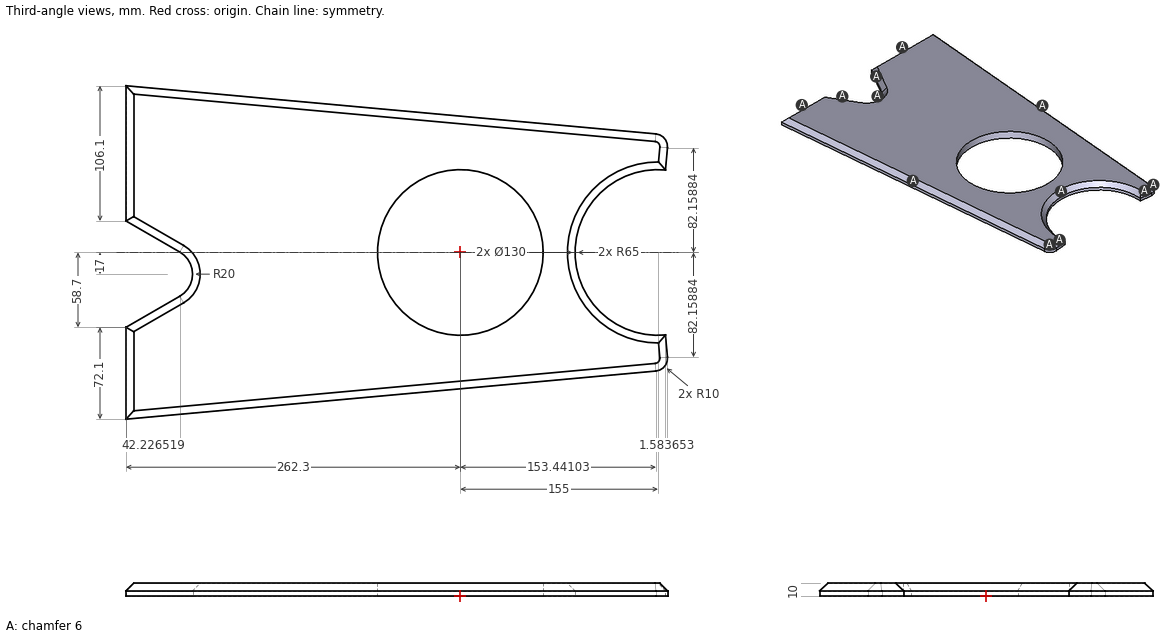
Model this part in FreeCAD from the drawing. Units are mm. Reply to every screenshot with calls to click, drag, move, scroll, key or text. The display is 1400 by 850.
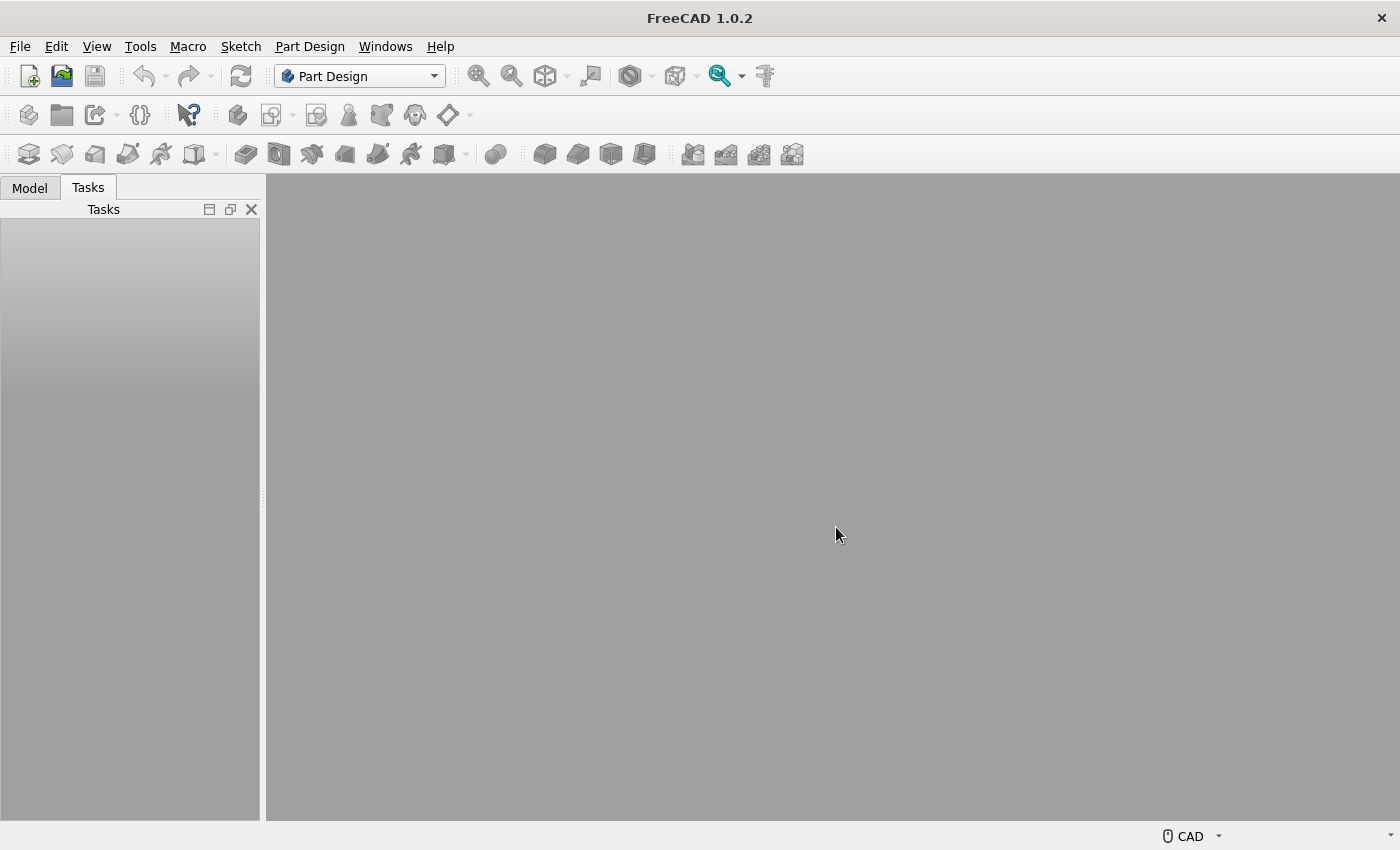
click(29, 76)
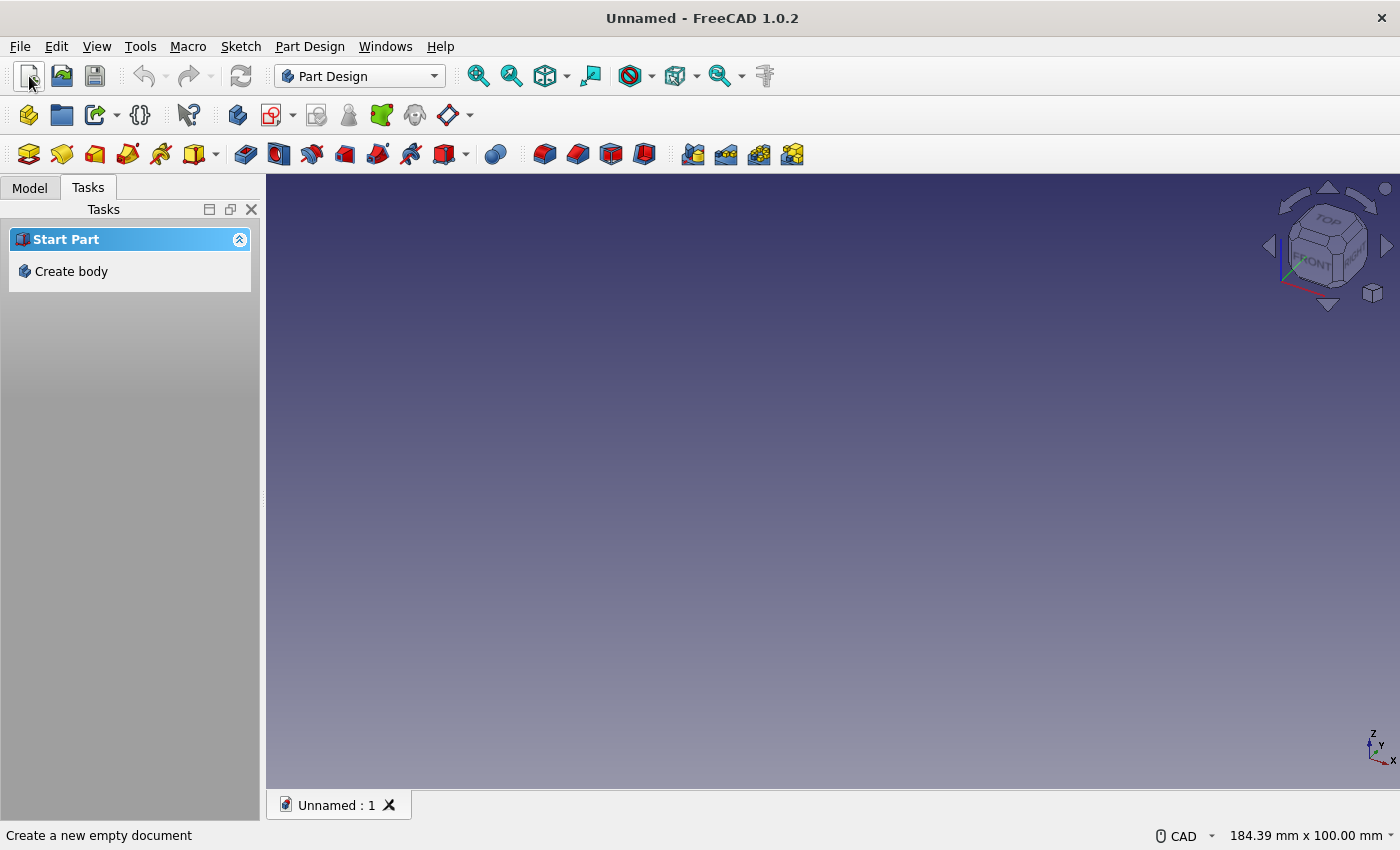
click(270, 116)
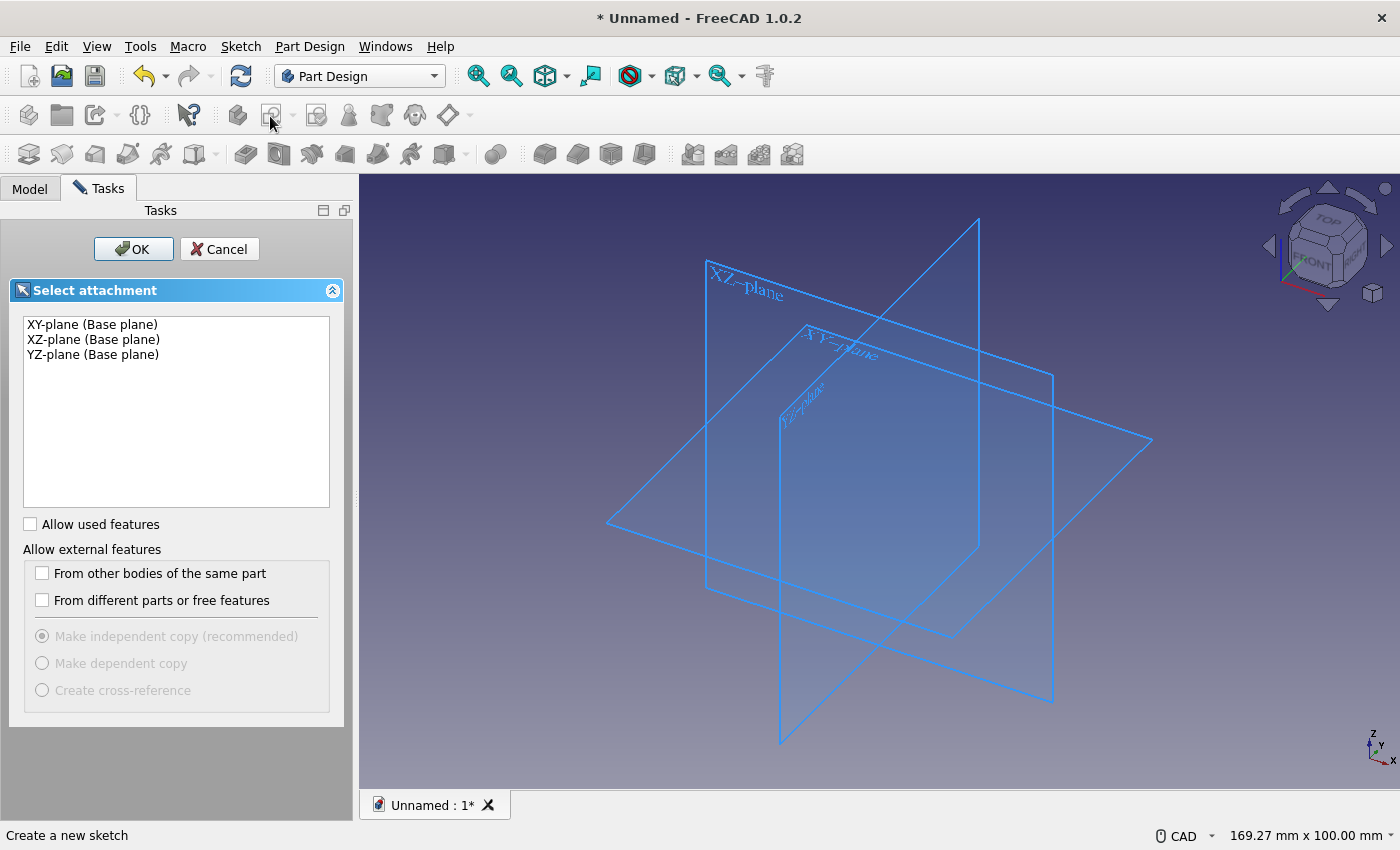
click(84, 324)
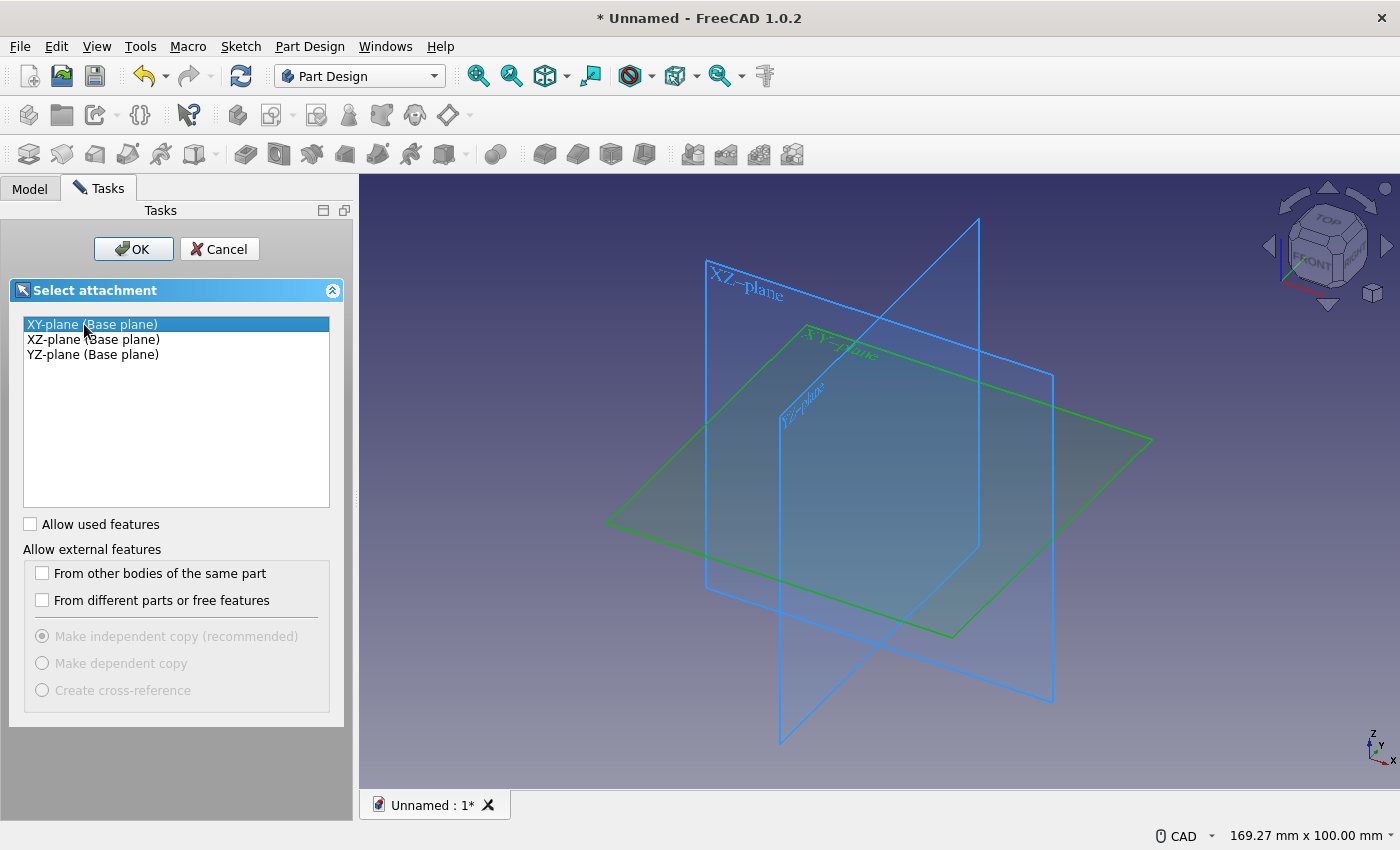
click(134, 249)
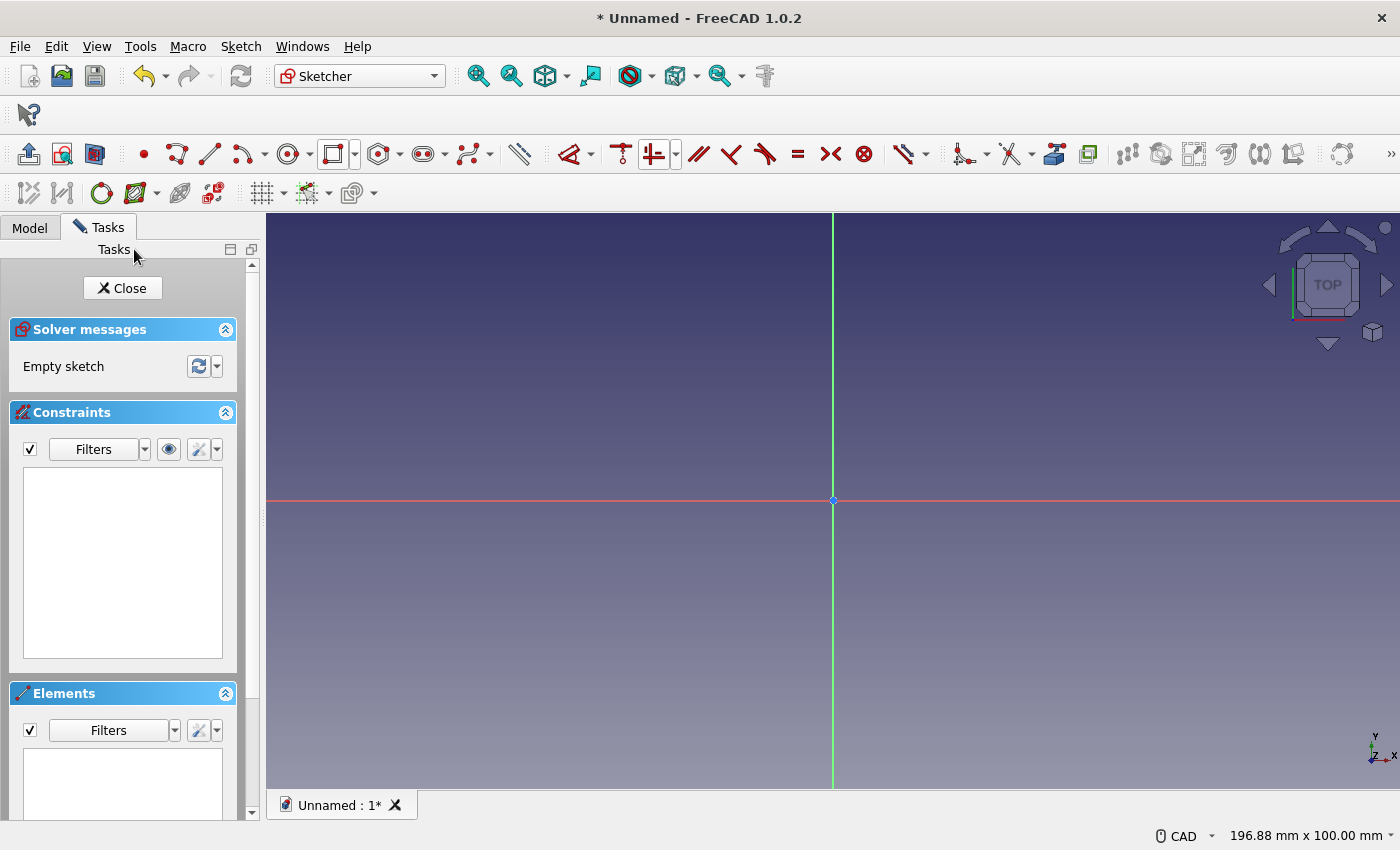
scroll(836, 501, down, 7)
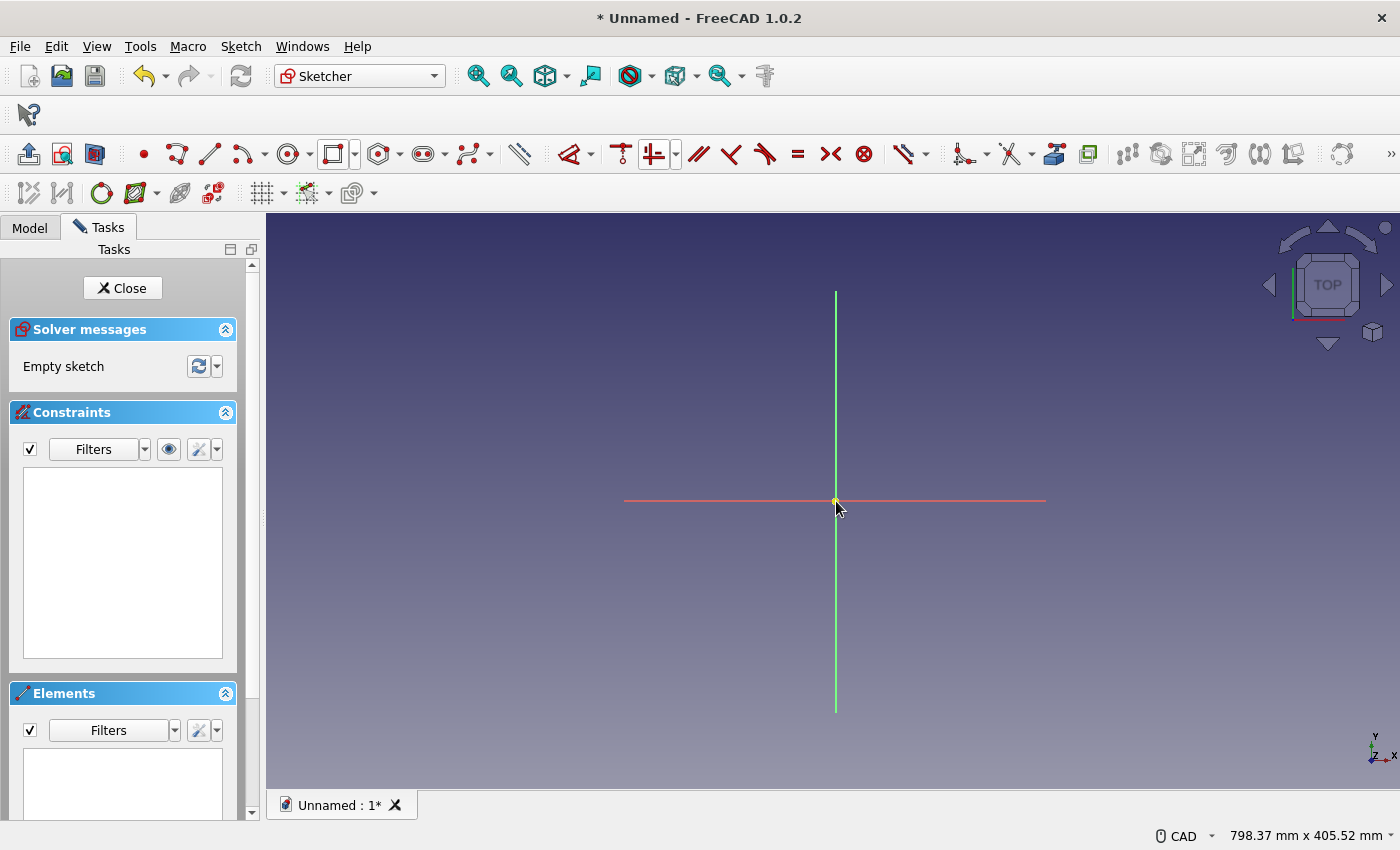
click(177, 154)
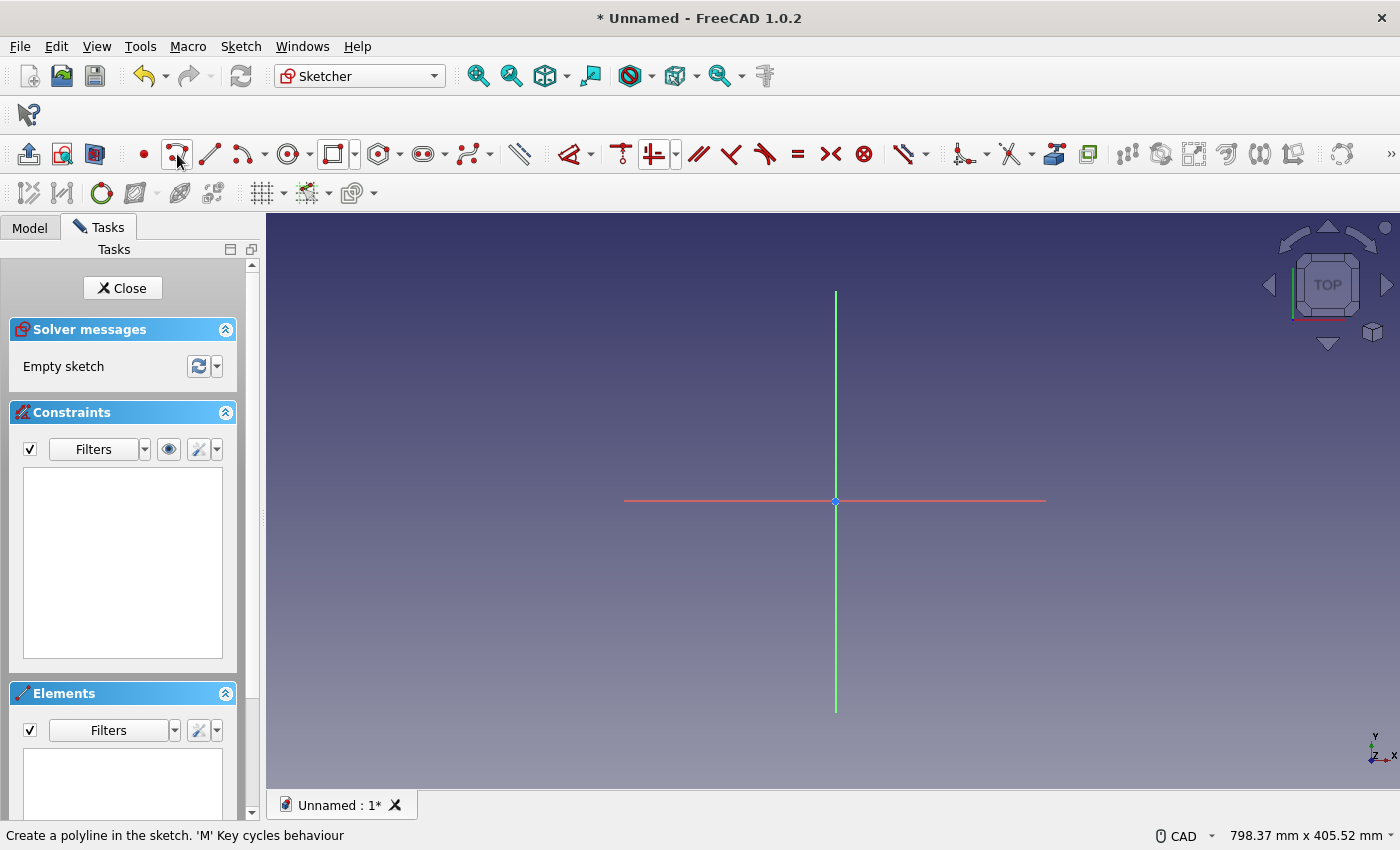
click(523, 550)
click(463, 585)
click(463, 687)
click(1054, 634)
right_click(1054, 634)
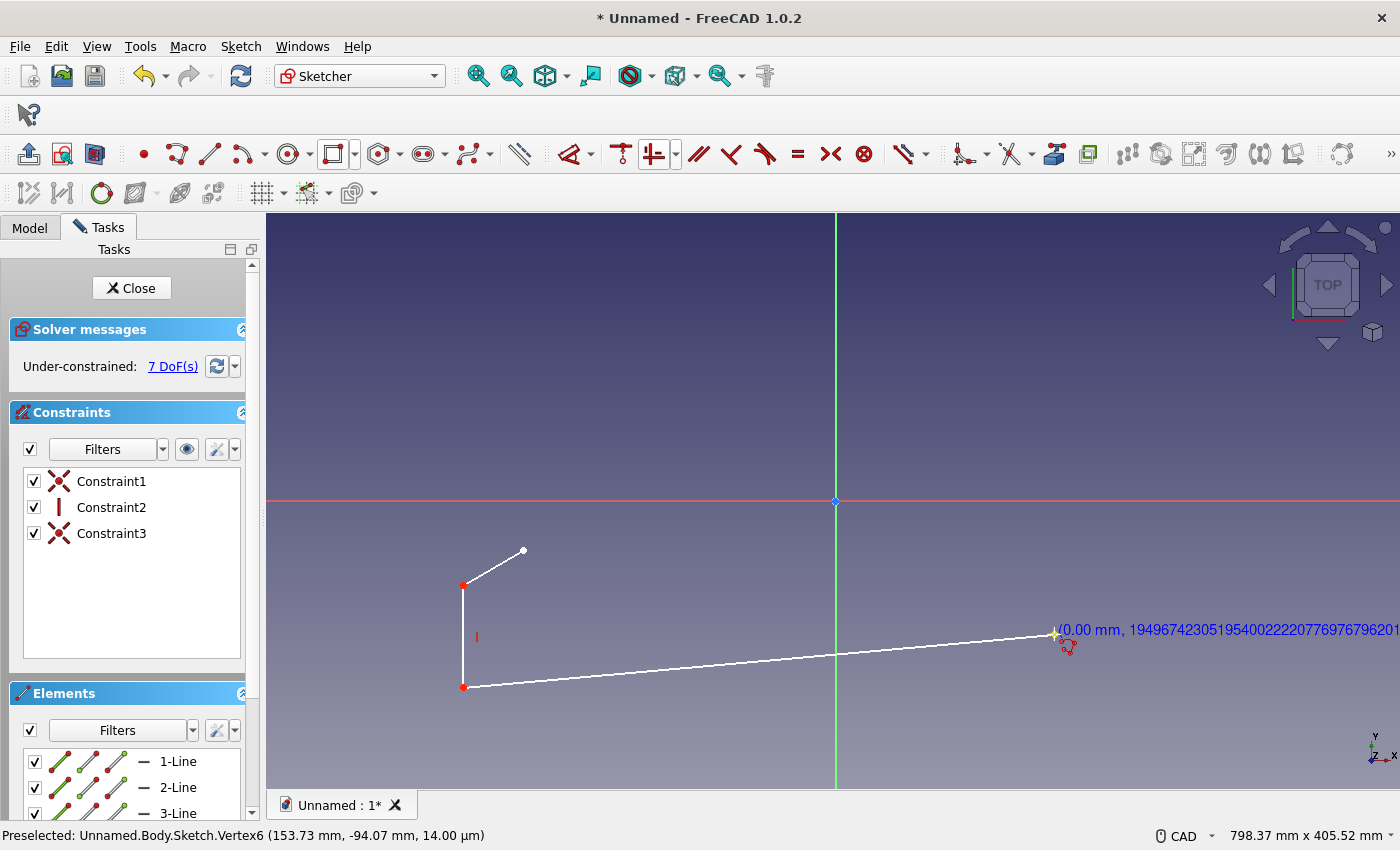
click(210, 154)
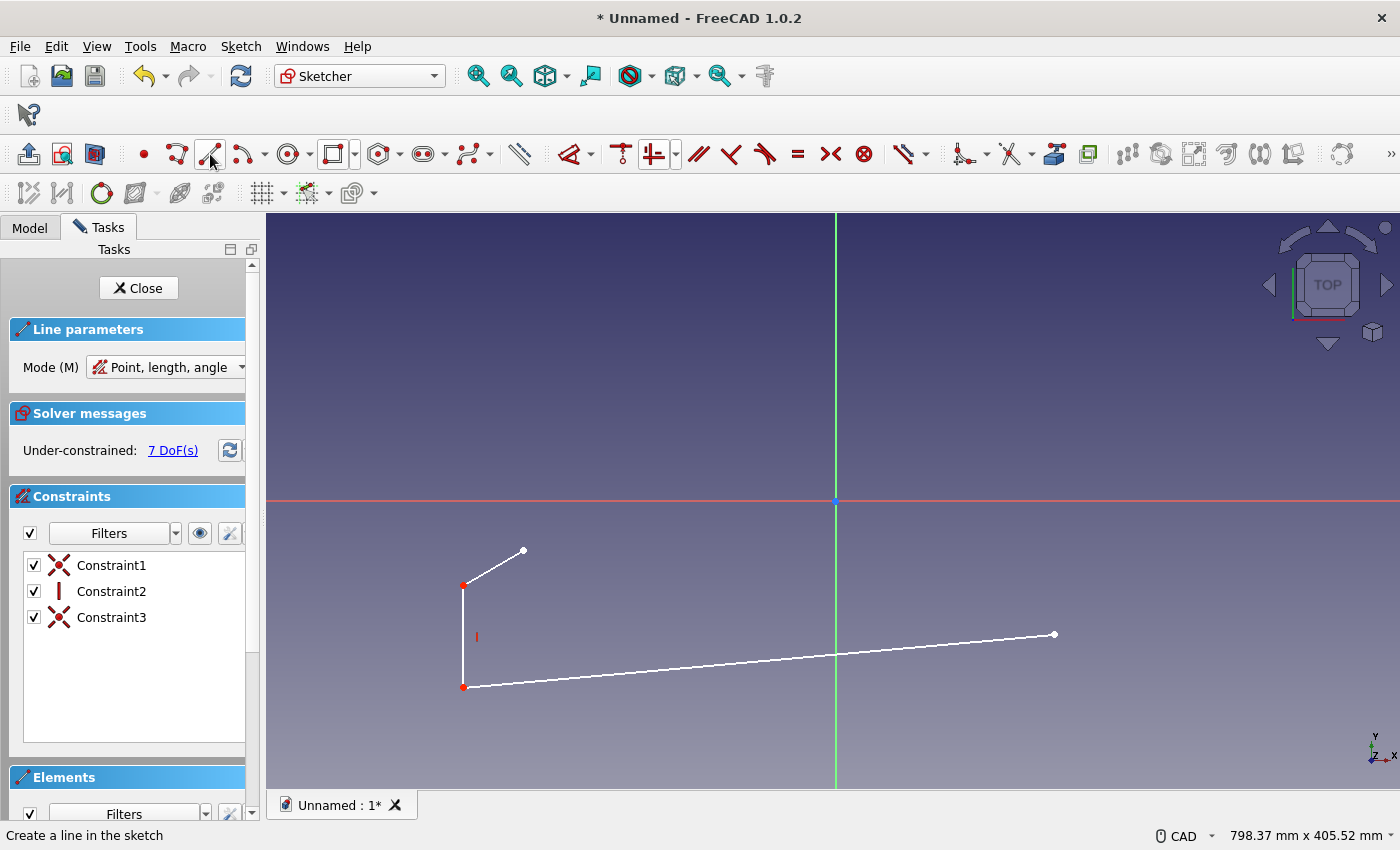
click(1066, 618)
click(1063, 593)